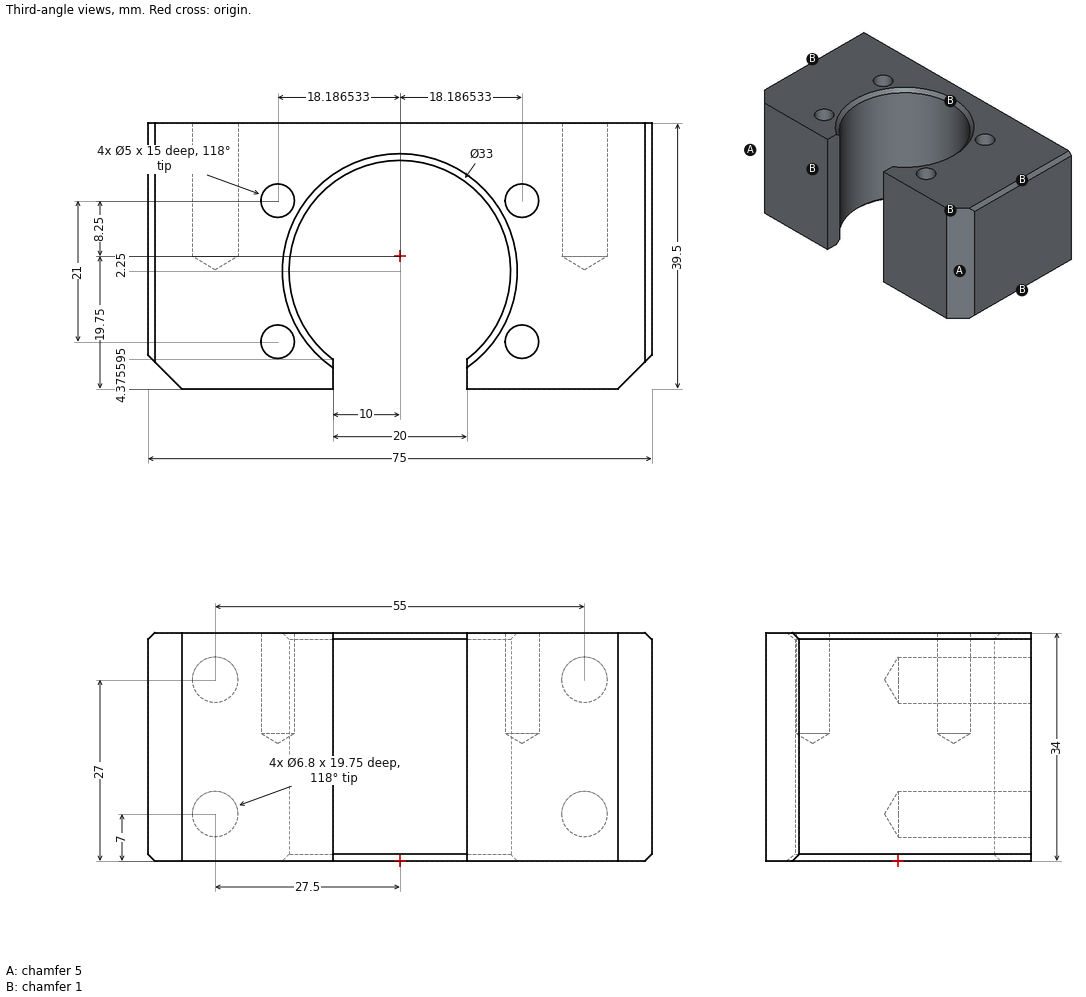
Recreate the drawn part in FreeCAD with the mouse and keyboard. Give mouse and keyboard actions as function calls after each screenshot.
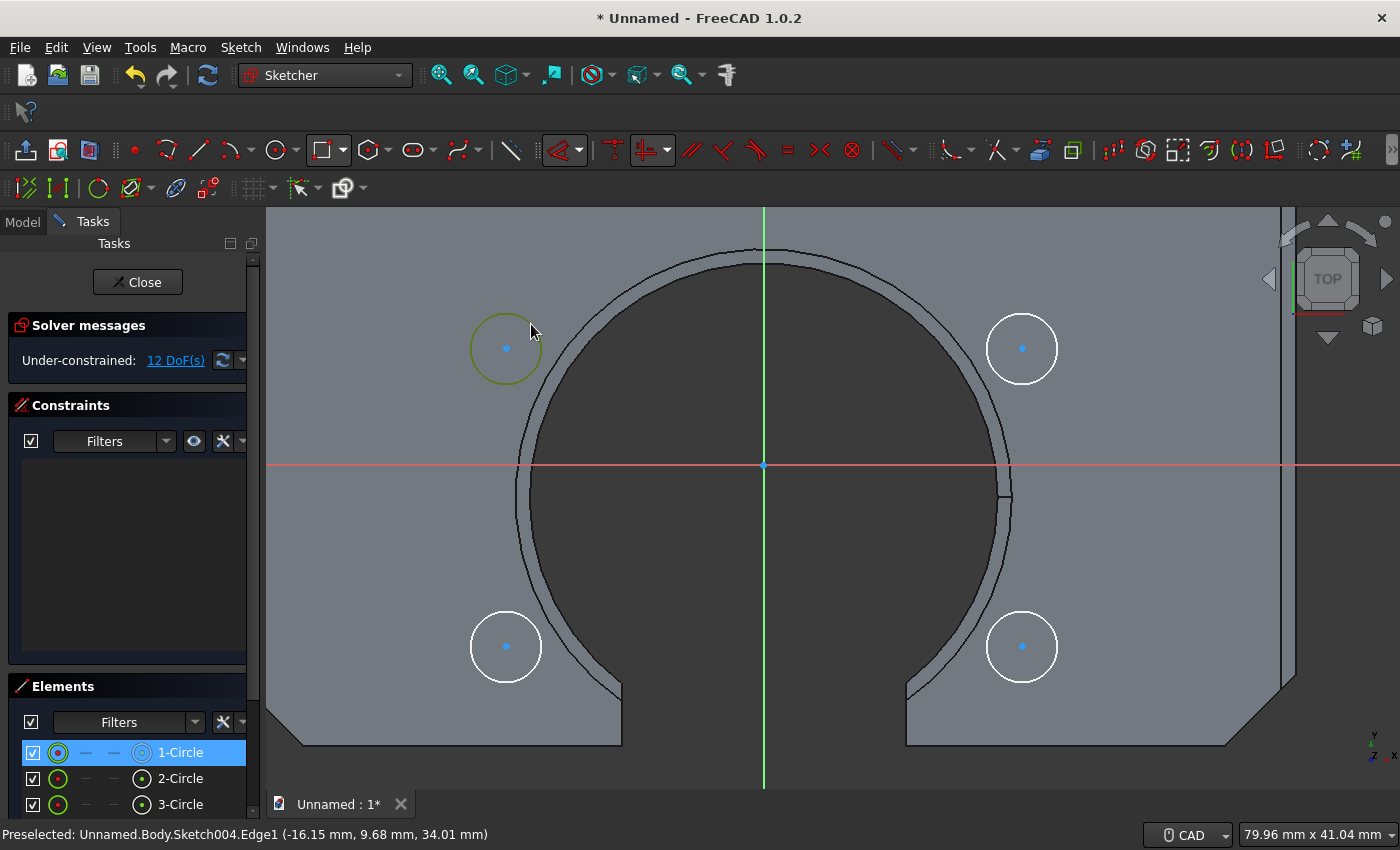
click(531, 622)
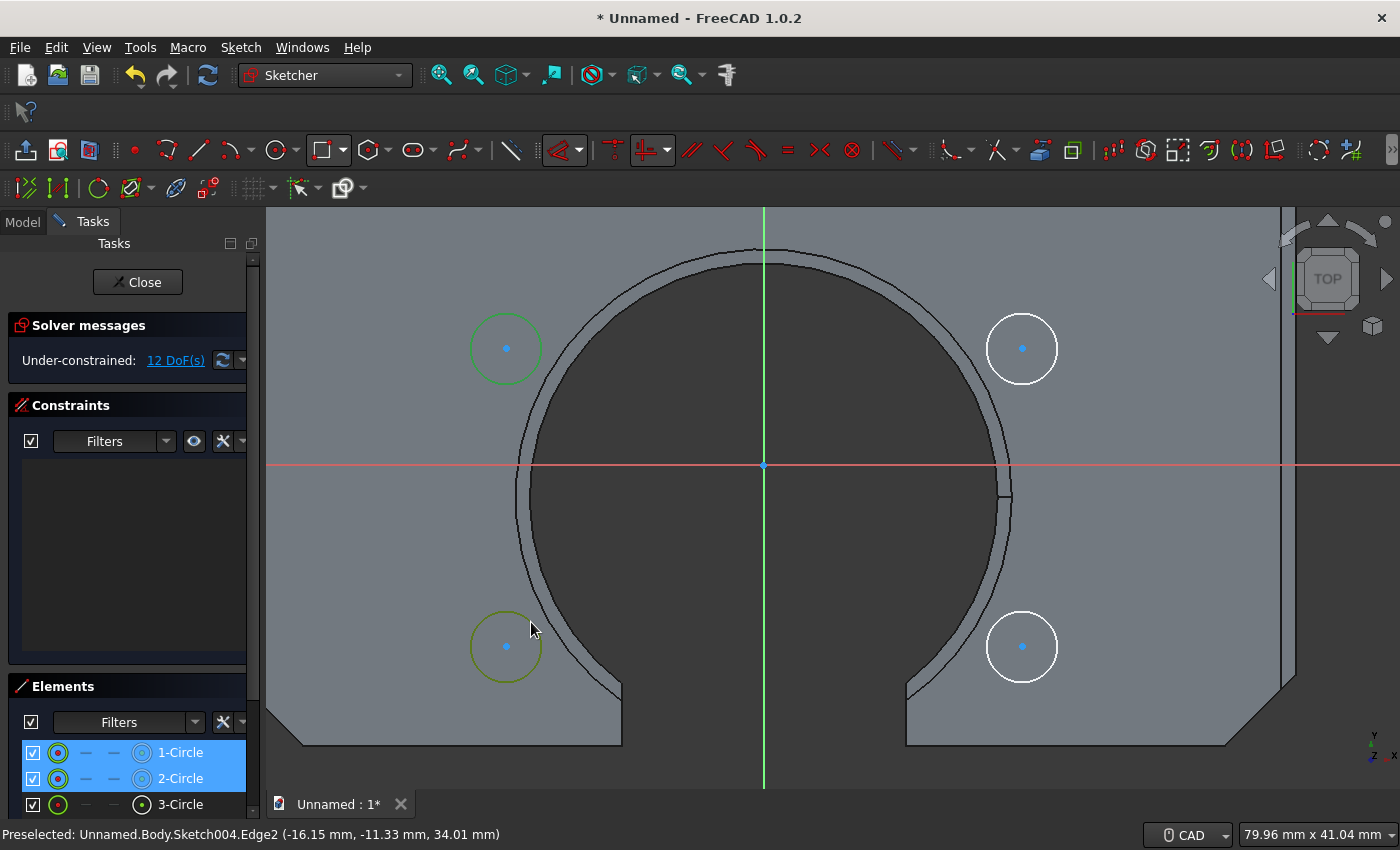
click(1047, 324)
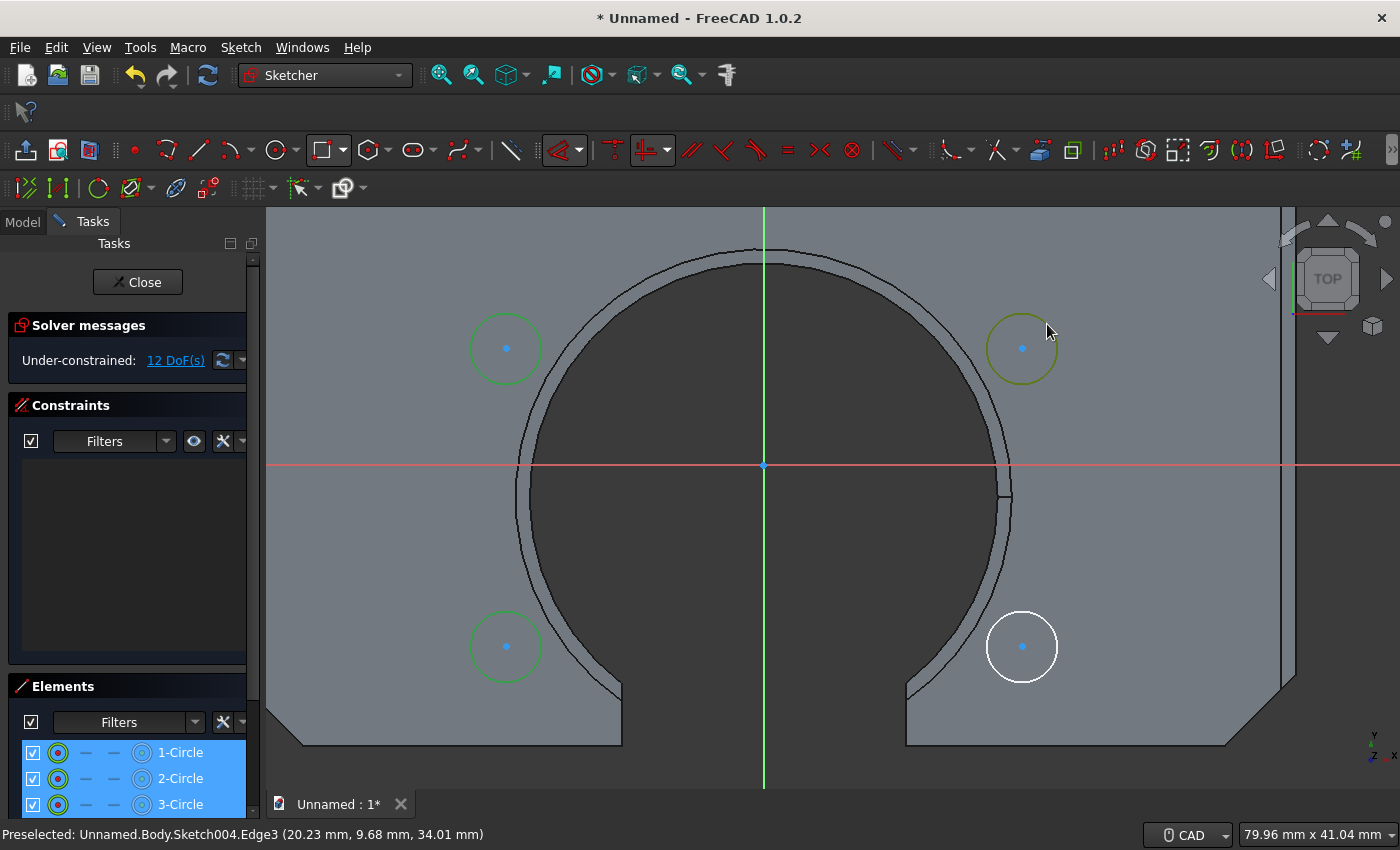
click(1047, 622)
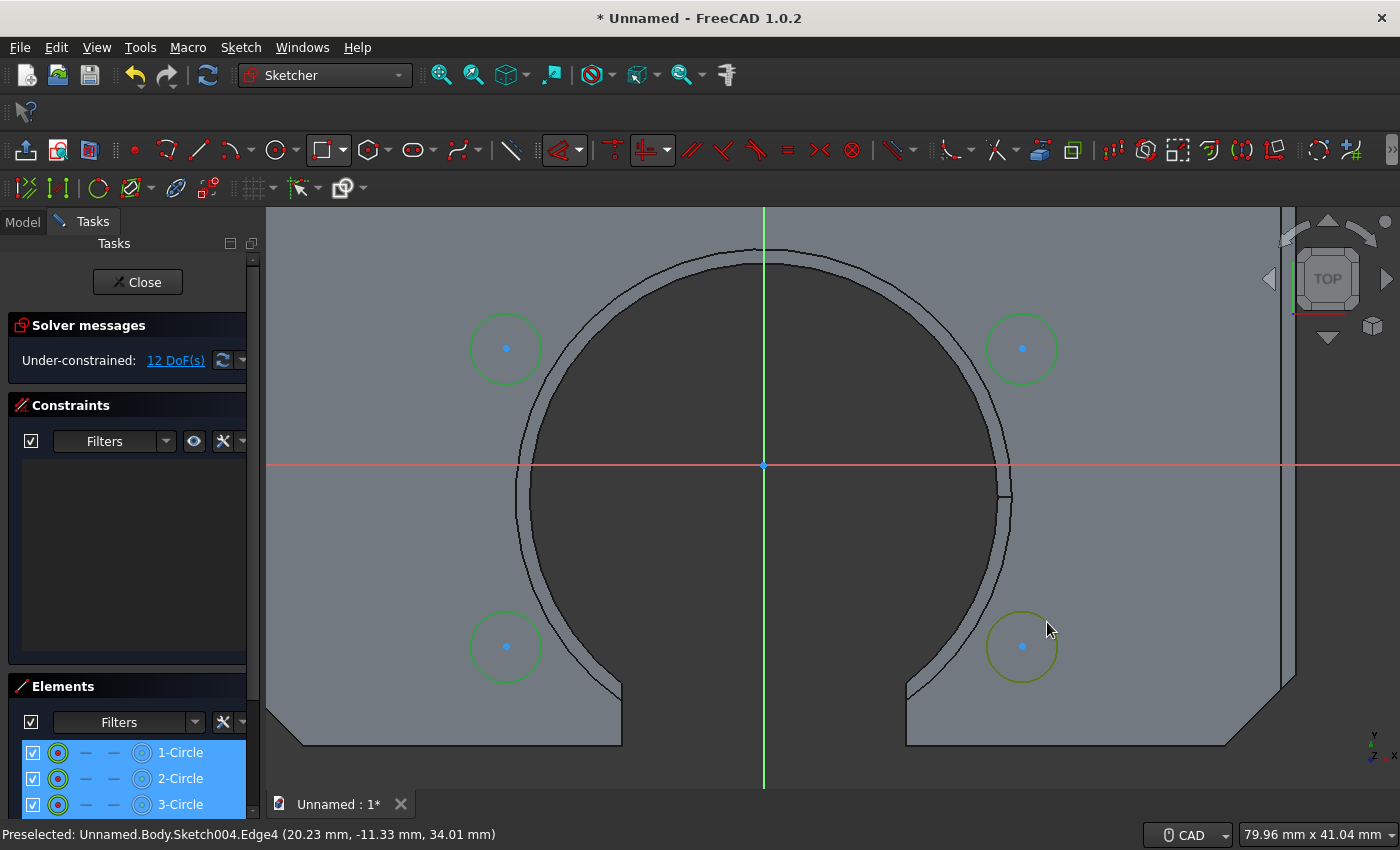
click(788, 150)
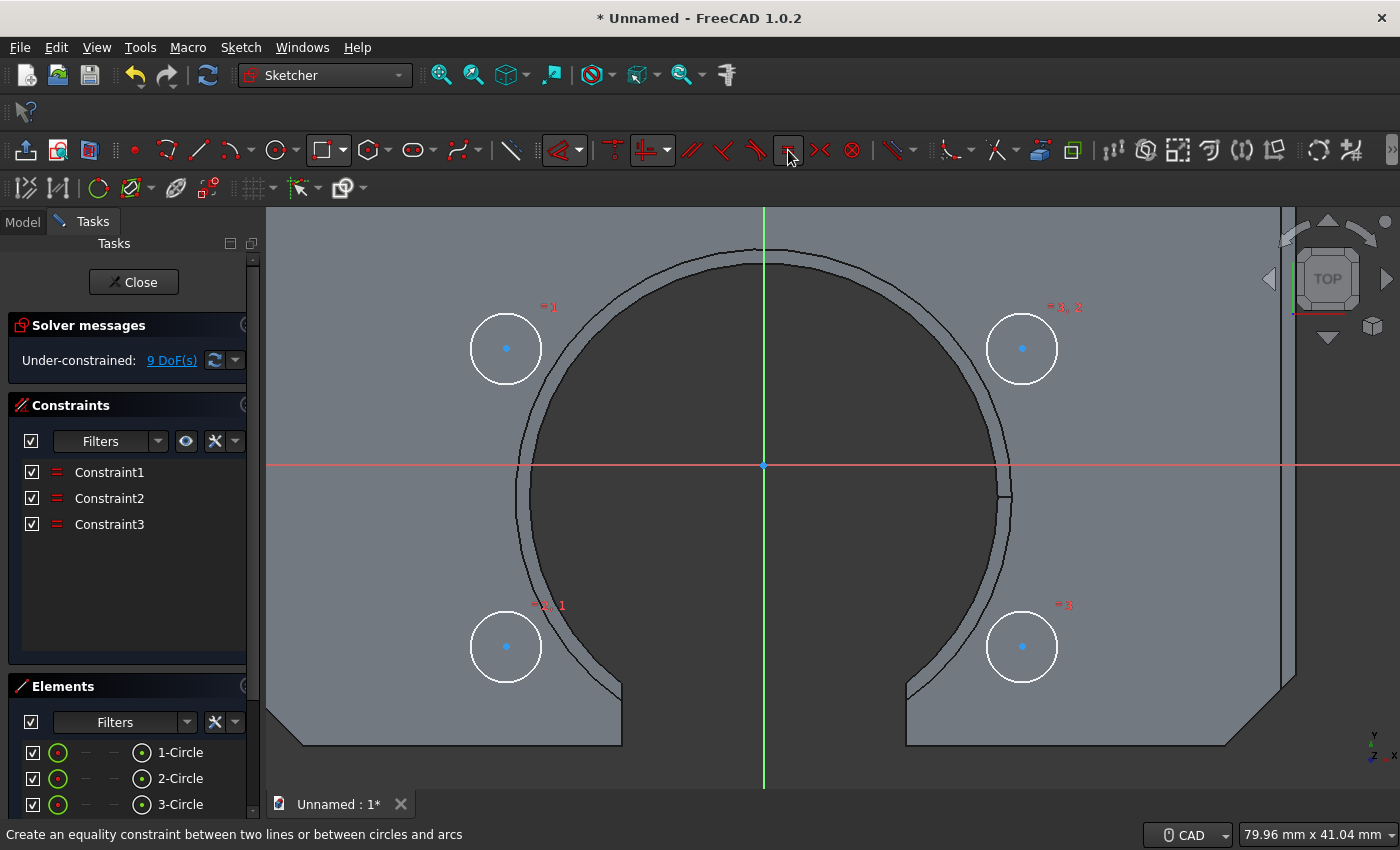
click(506, 349)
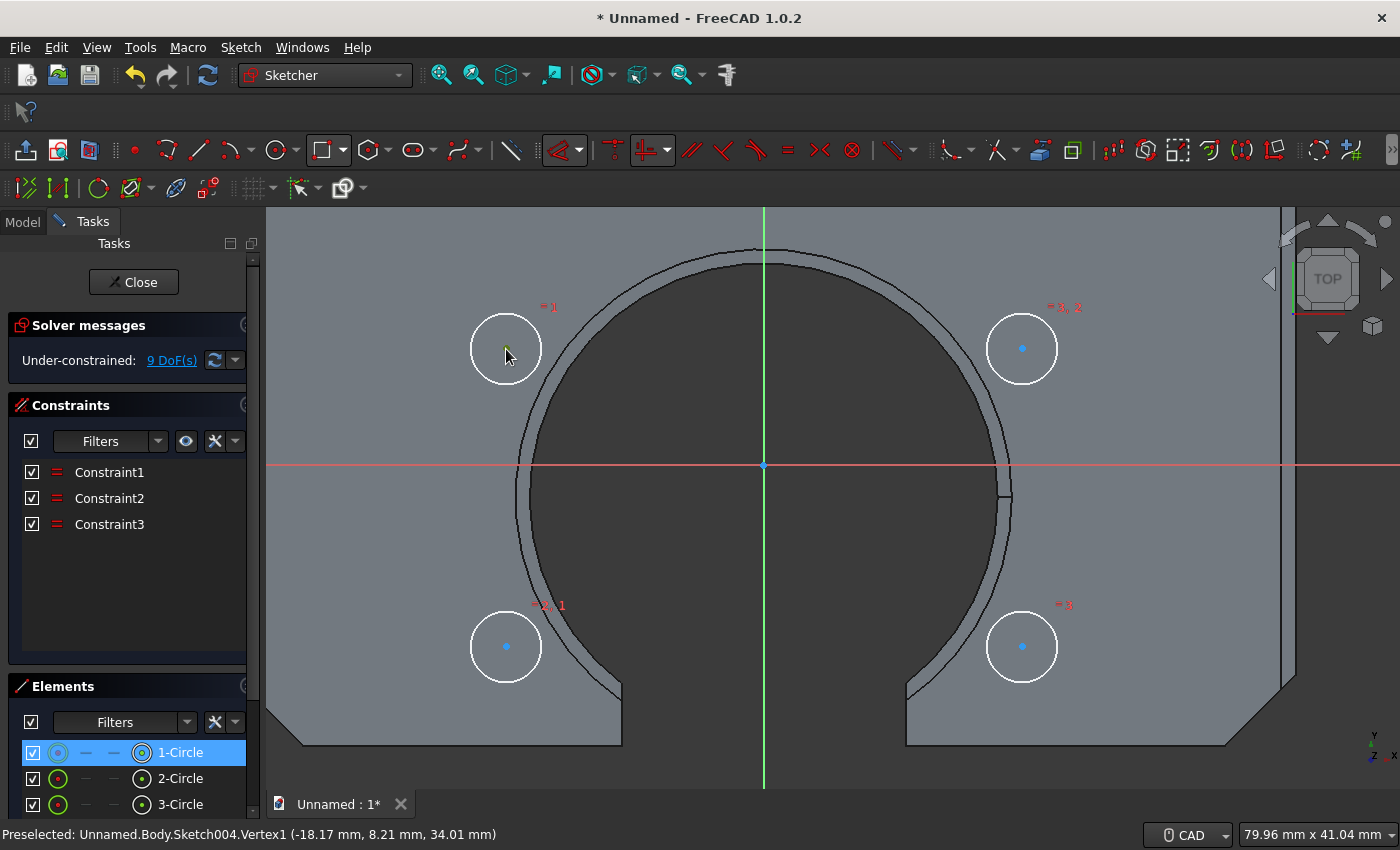
click(506, 647)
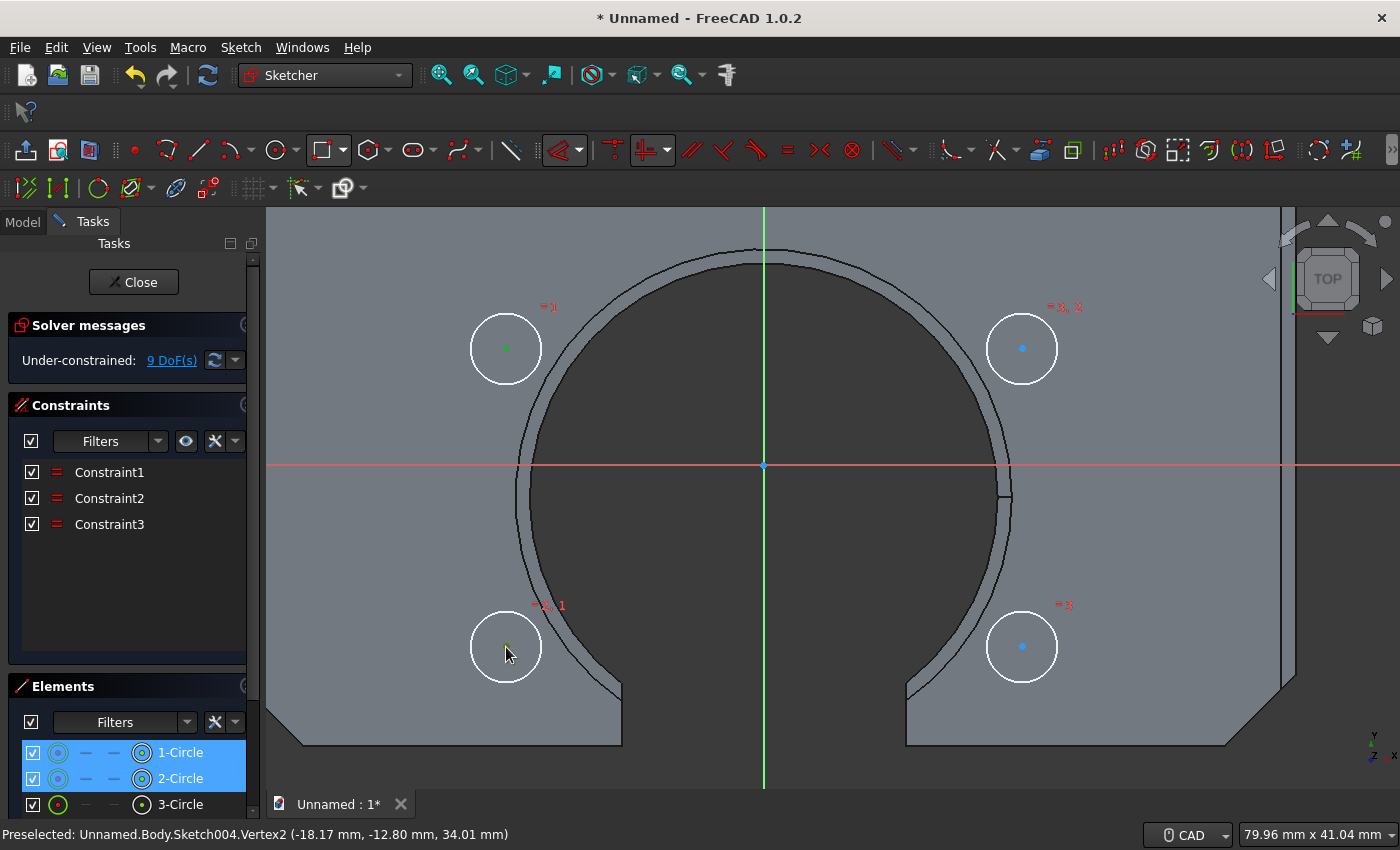
click(670, 150)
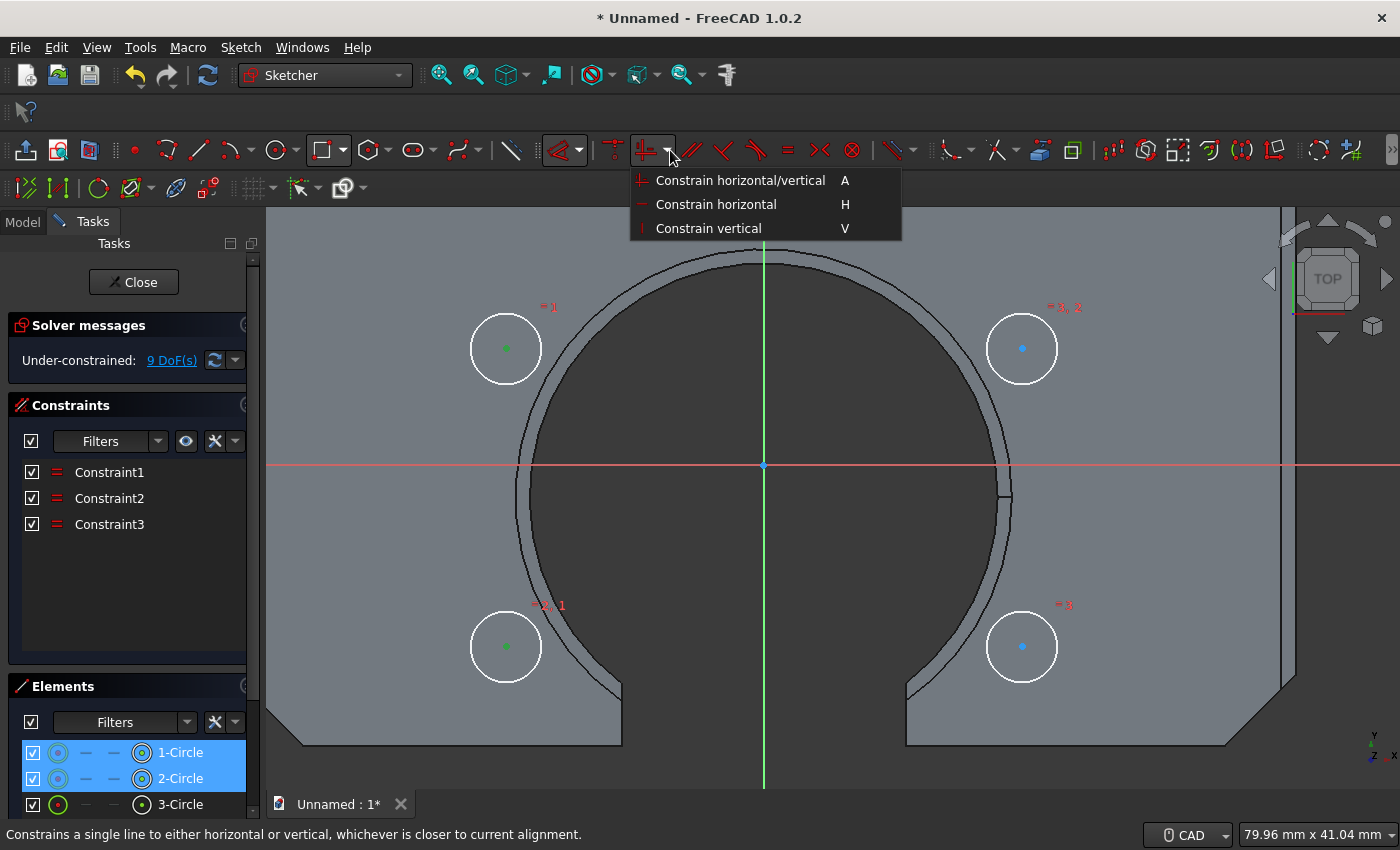
click(766, 228)